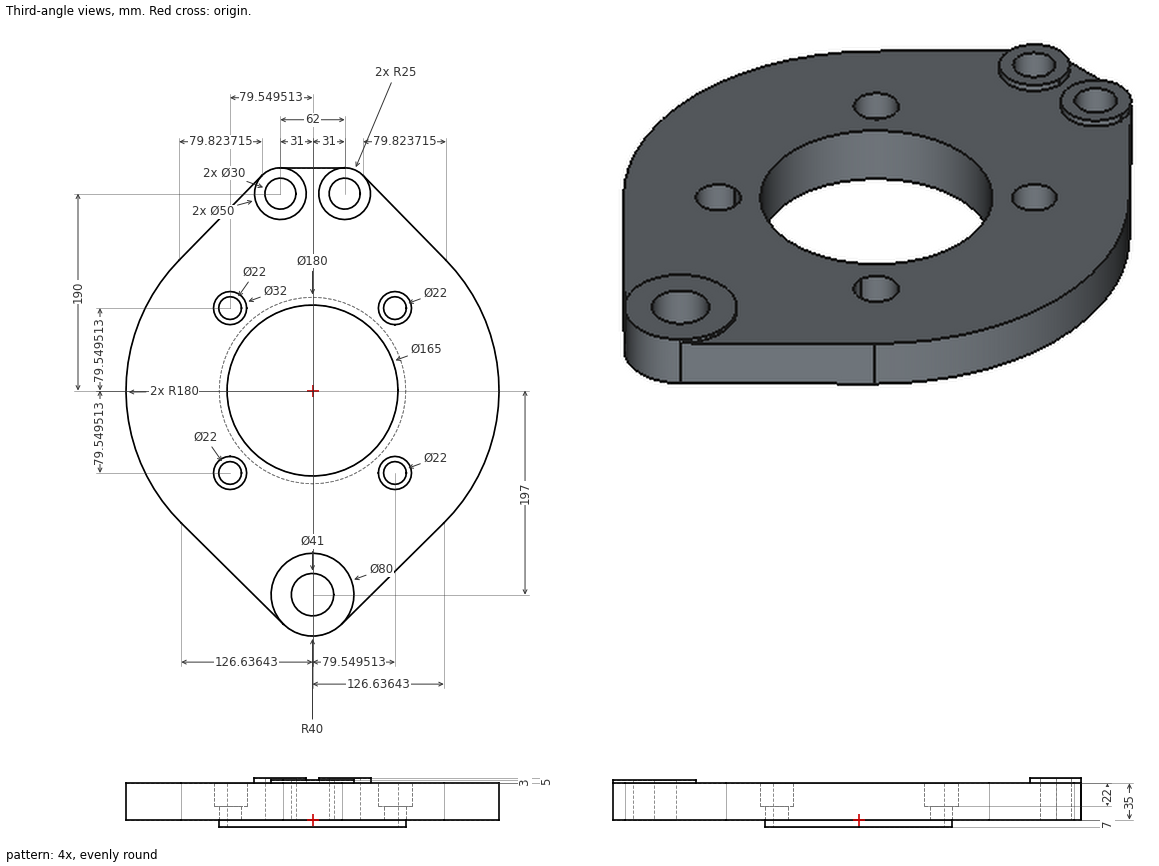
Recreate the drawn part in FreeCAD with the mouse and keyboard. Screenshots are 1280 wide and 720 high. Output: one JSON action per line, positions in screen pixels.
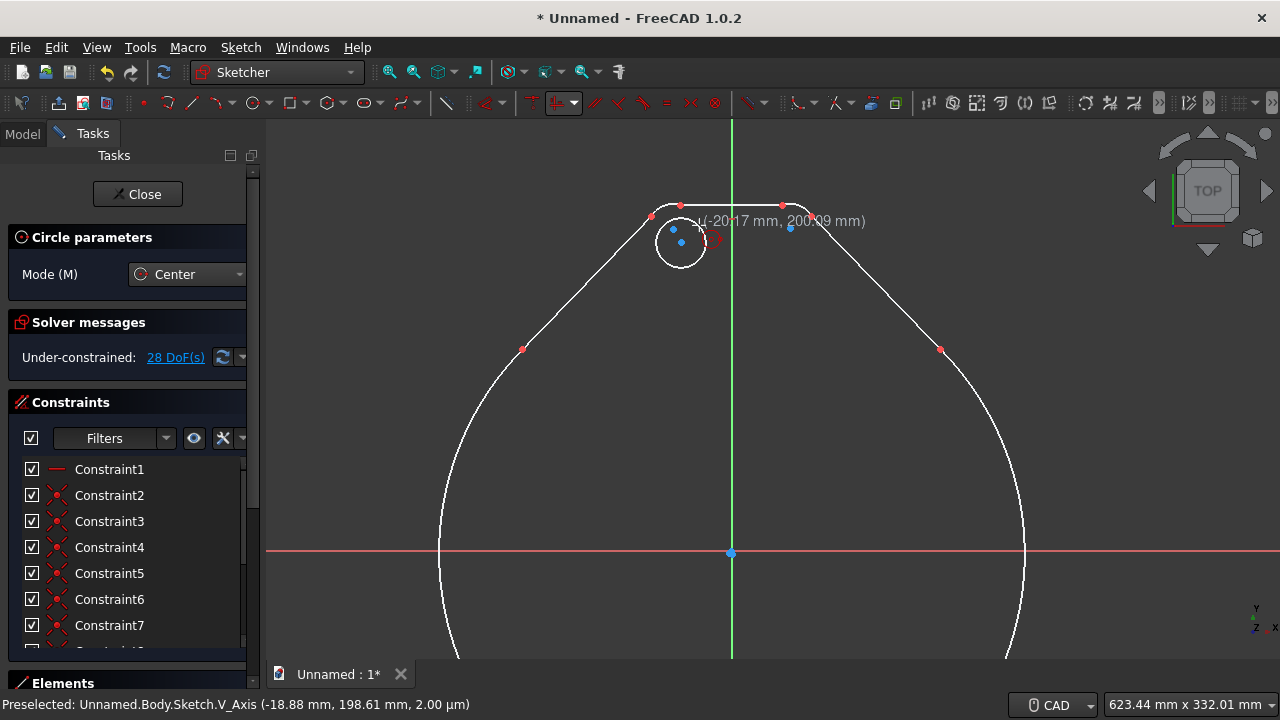
{"action": "left_click", "coordinate": [732, 551]}
{"action": "left_click", "coordinate": [827, 457]}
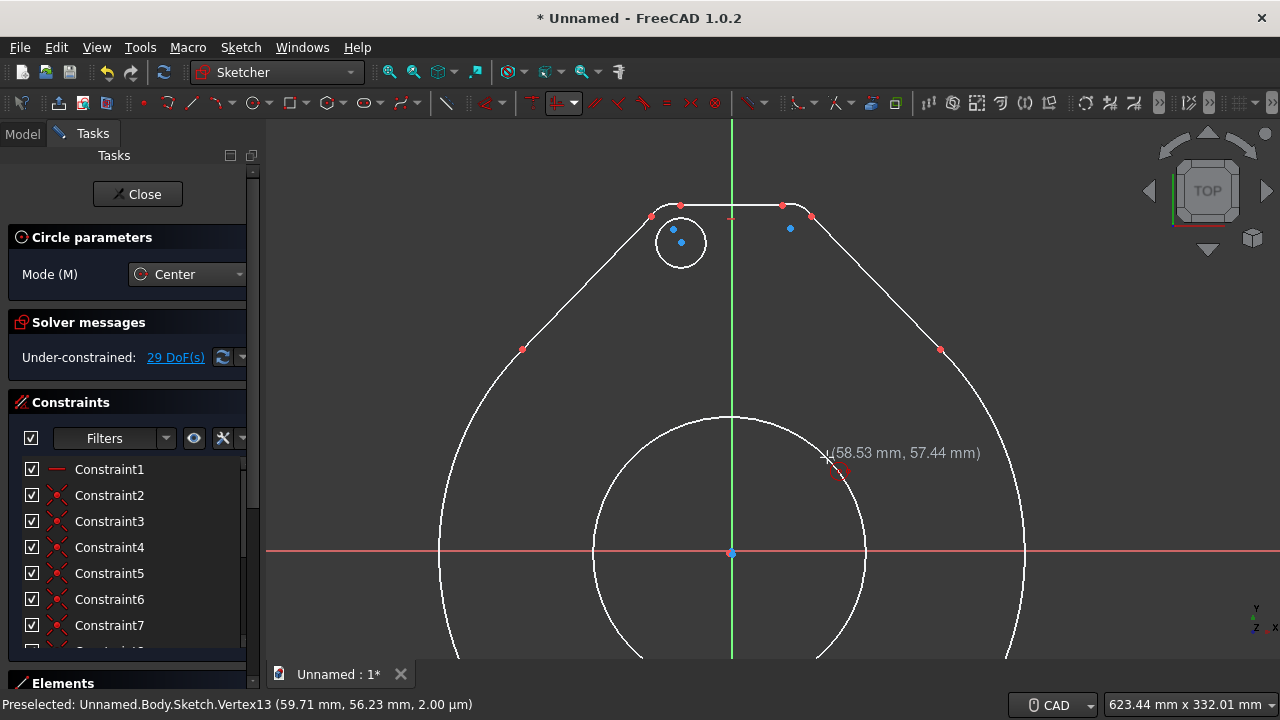
{"action": "left_click", "coordinate": [782, 242]}
{"action": "left_click", "coordinate": [799, 225]}
{"action": "key", "text": "Escape"}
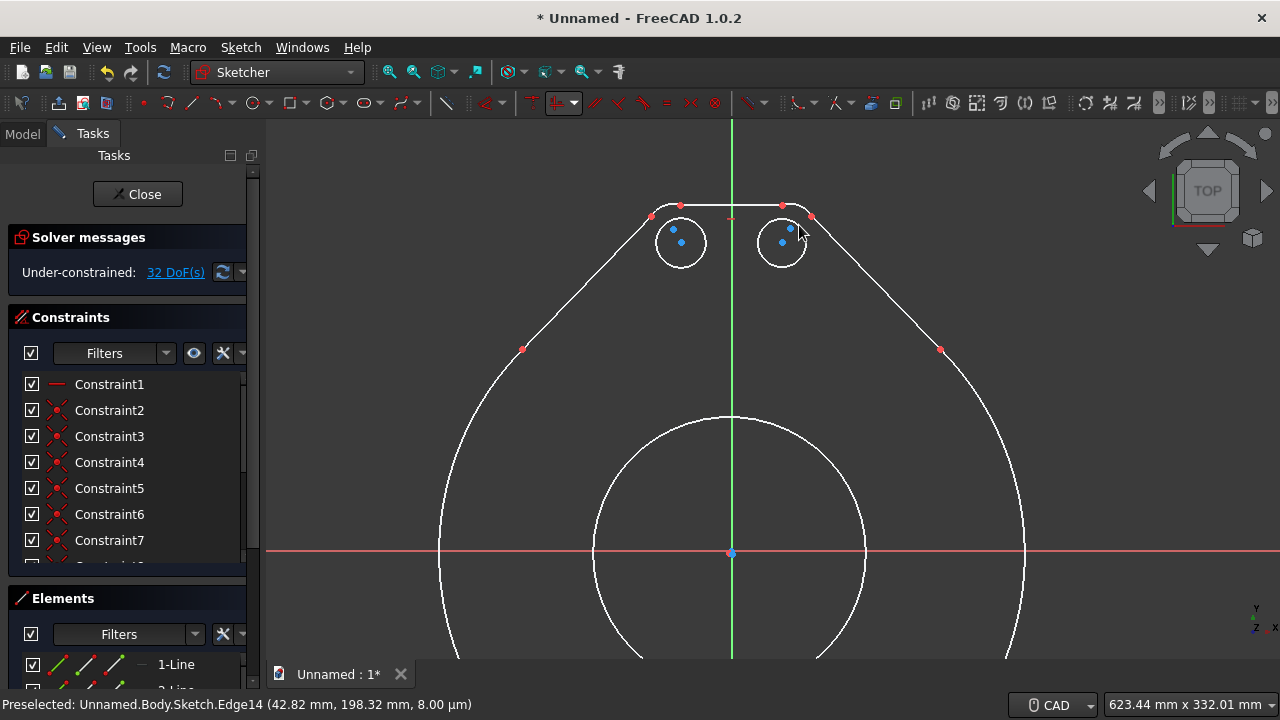
{"action": "left_click", "coordinate": [613, 256]}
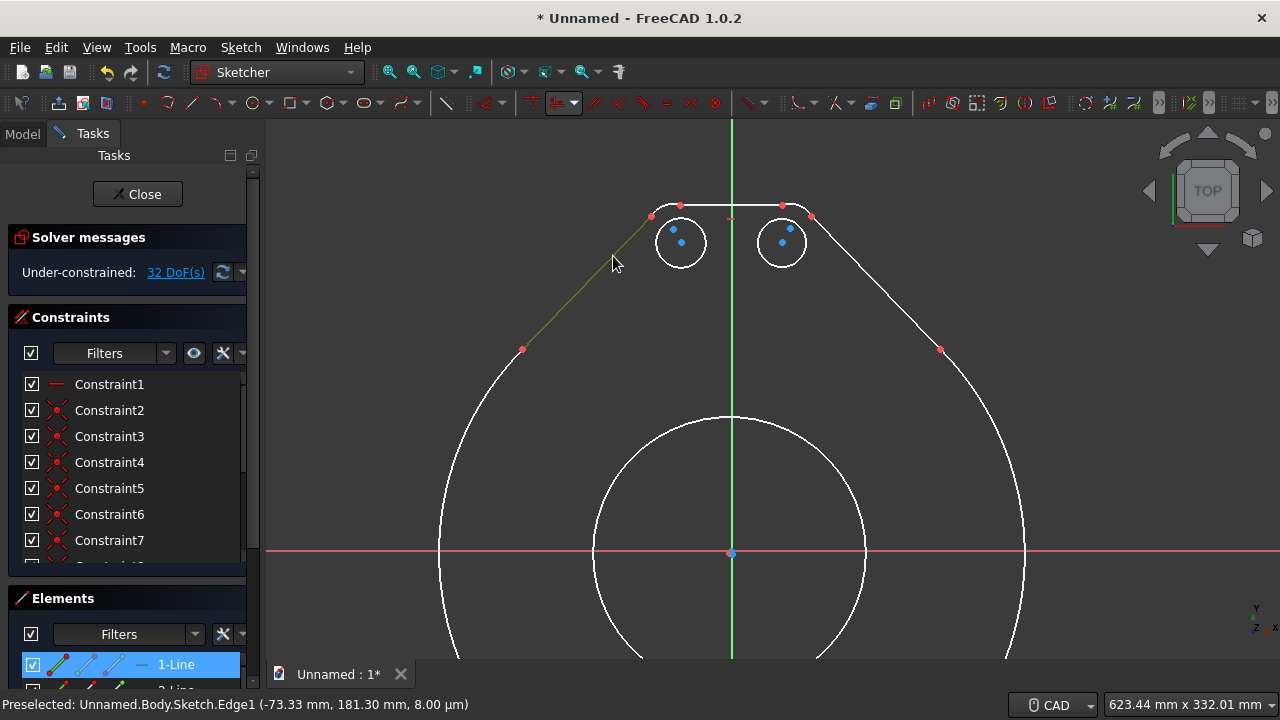
{"action": "scroll", "coordinate": [671, 204], "scroll_direction": "up", "scroll_amount": 2}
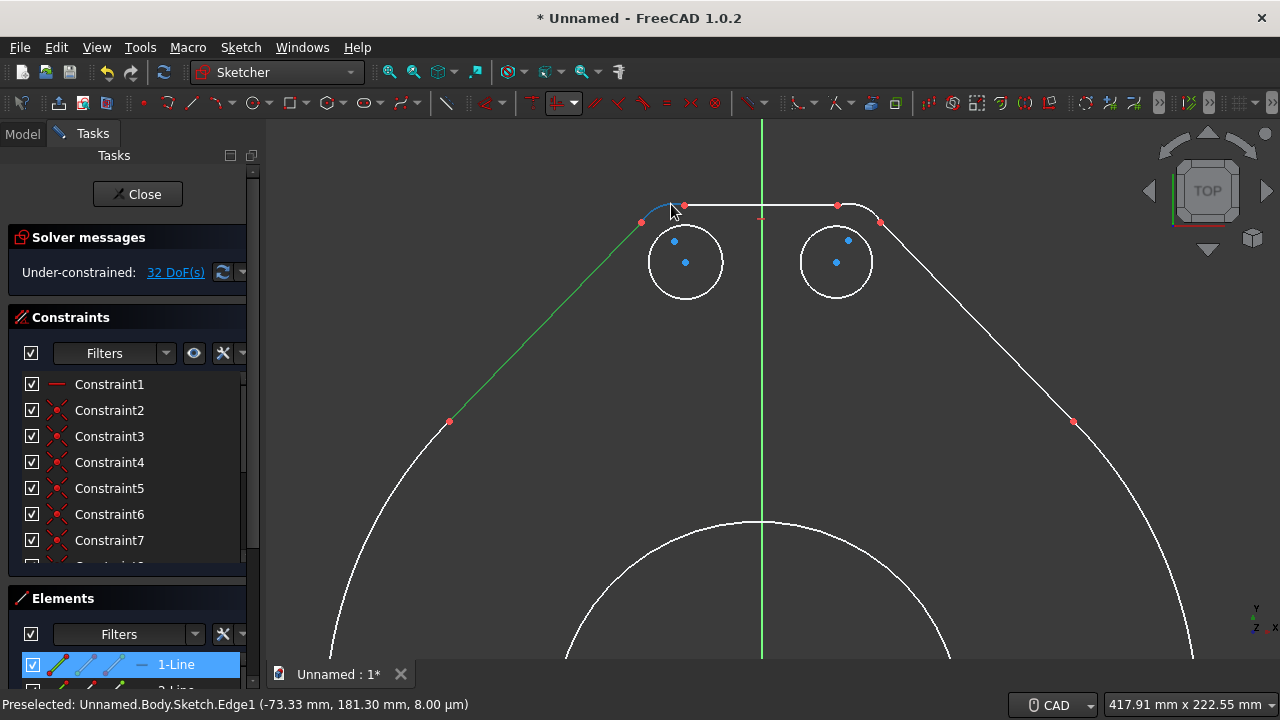
{"action": "left_click", "coordinate": [670, 204]}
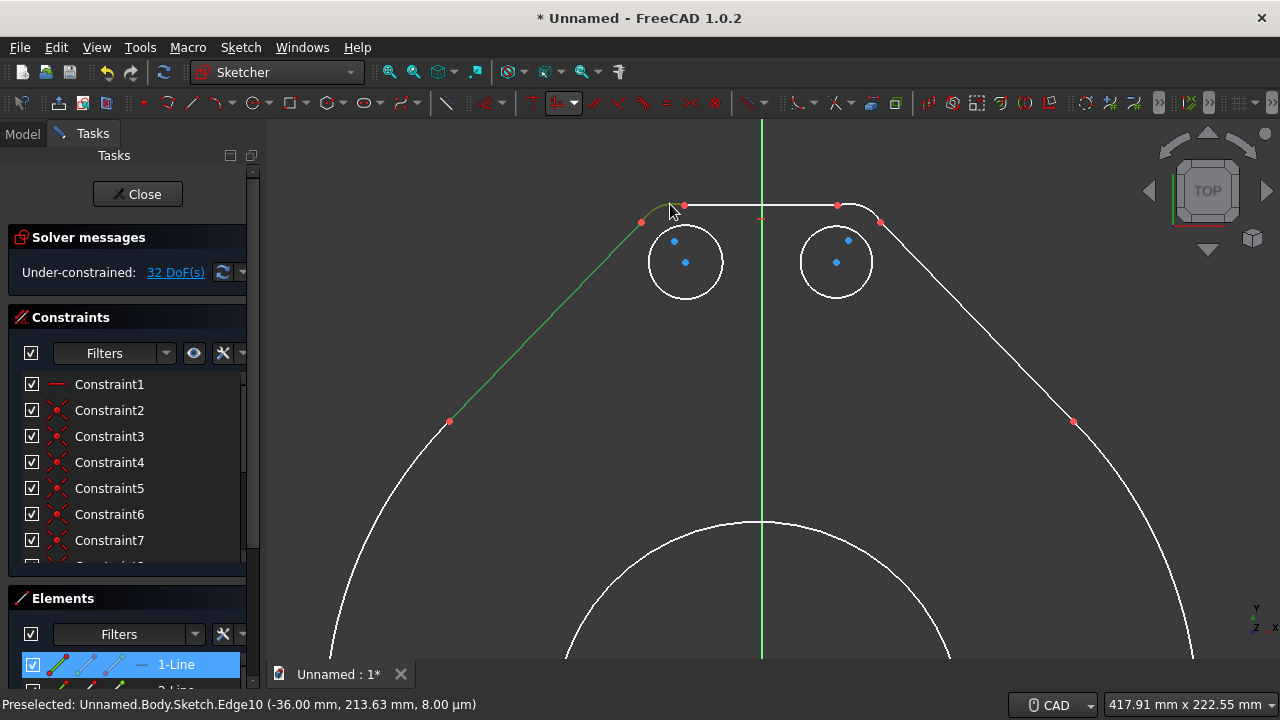
{"action": "left_click", "coordinate": [644, 104]}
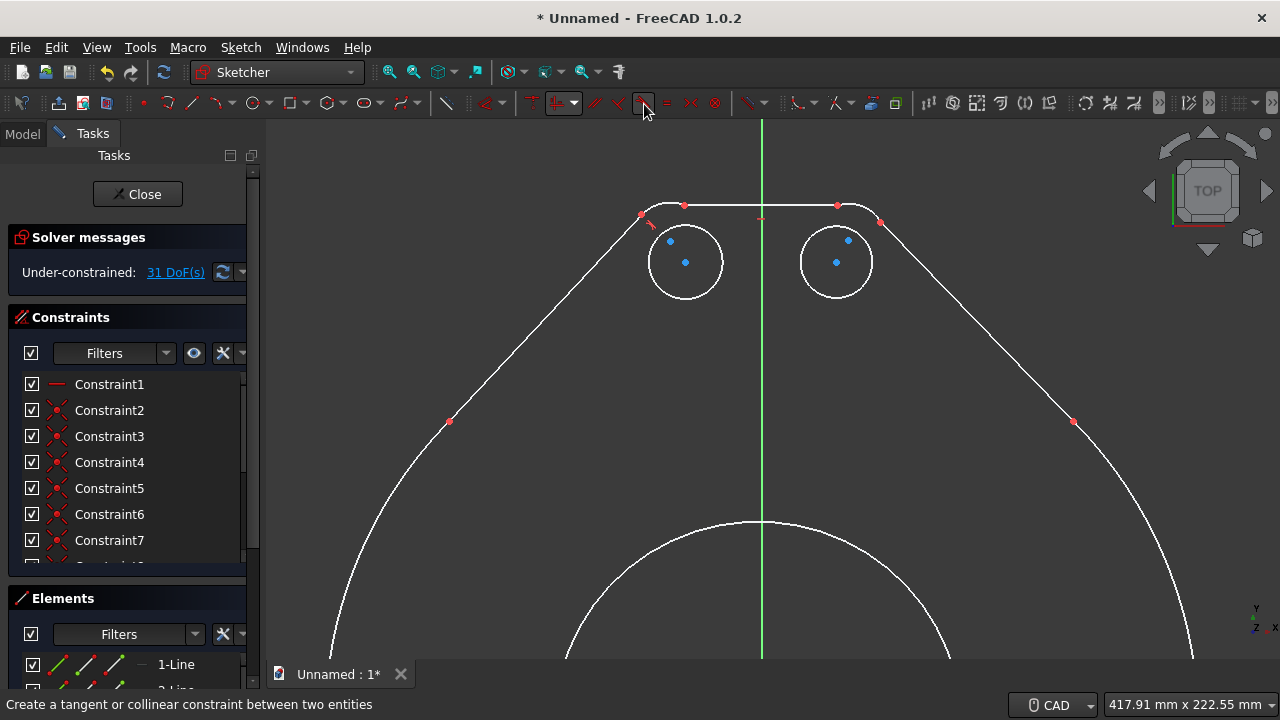
{"action": "scroll", "coordinate": [680, 234], "scroll_direction": "down", "scroll_amount": 6}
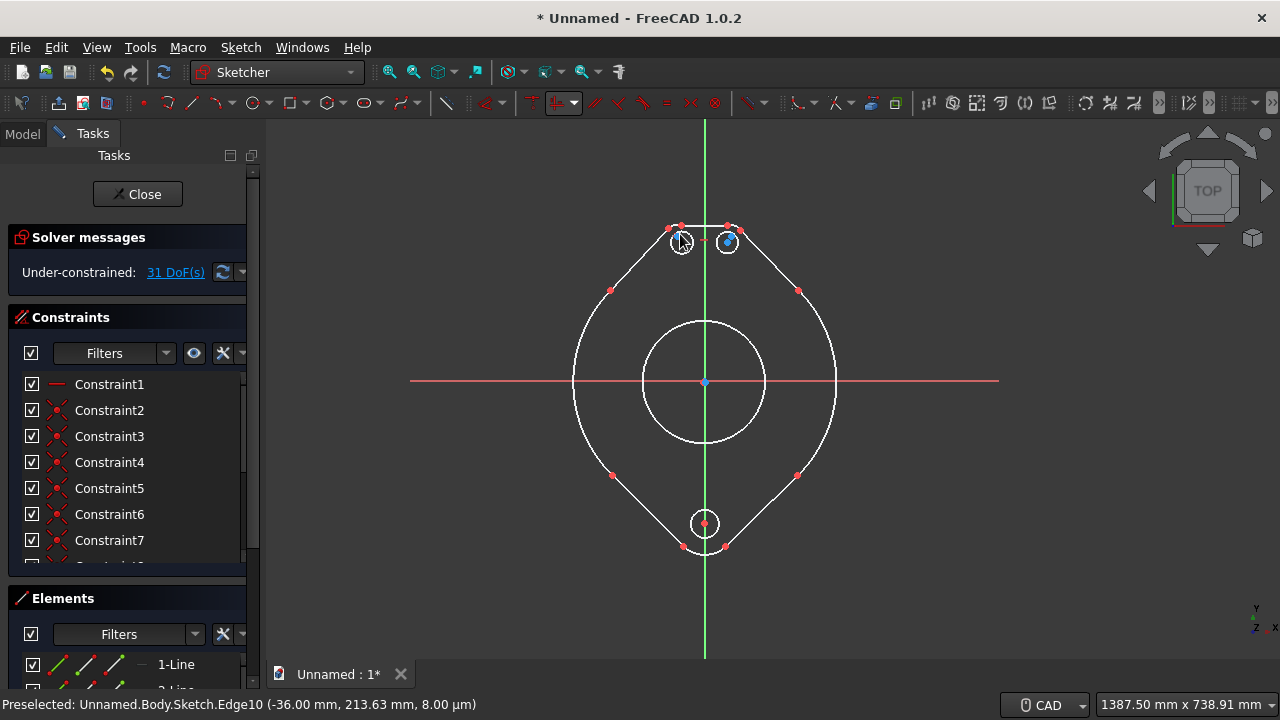
{"action": "left_click", "coordinate": [634, 497]}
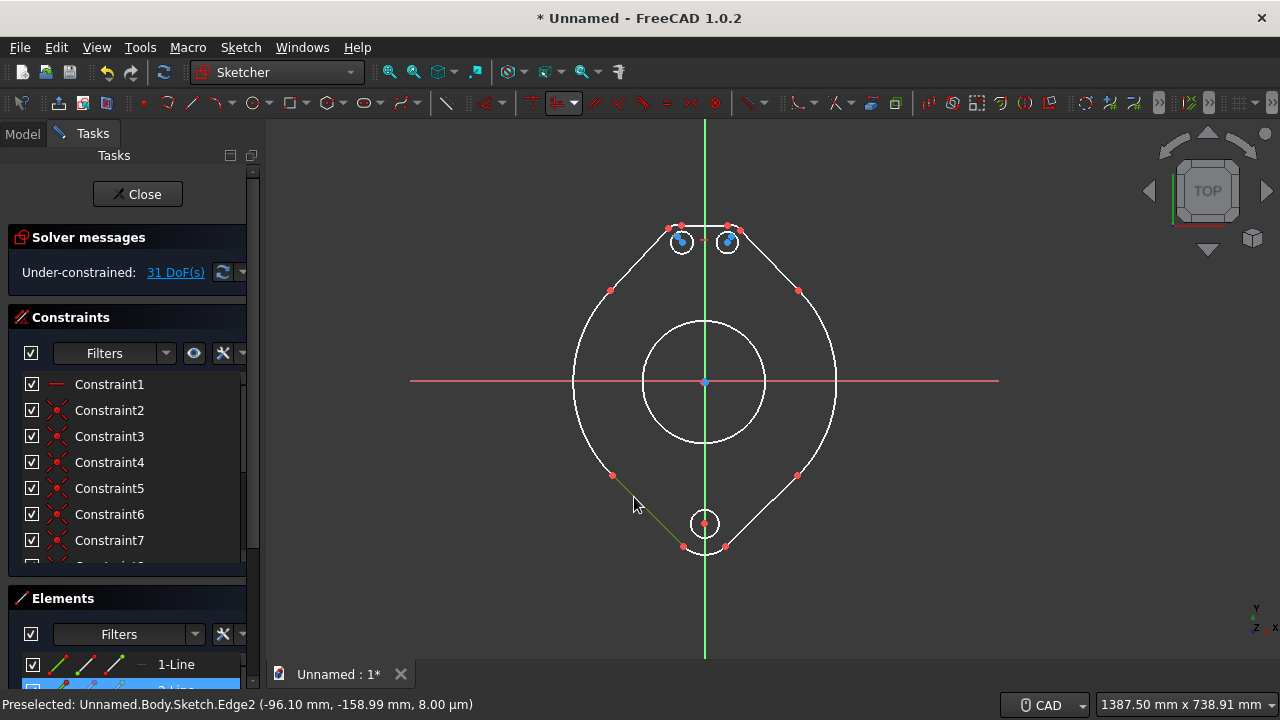
{"action": "scroll", "coordinate": [696, 553], "scroll_direction": "up", "scroll_amount": 3}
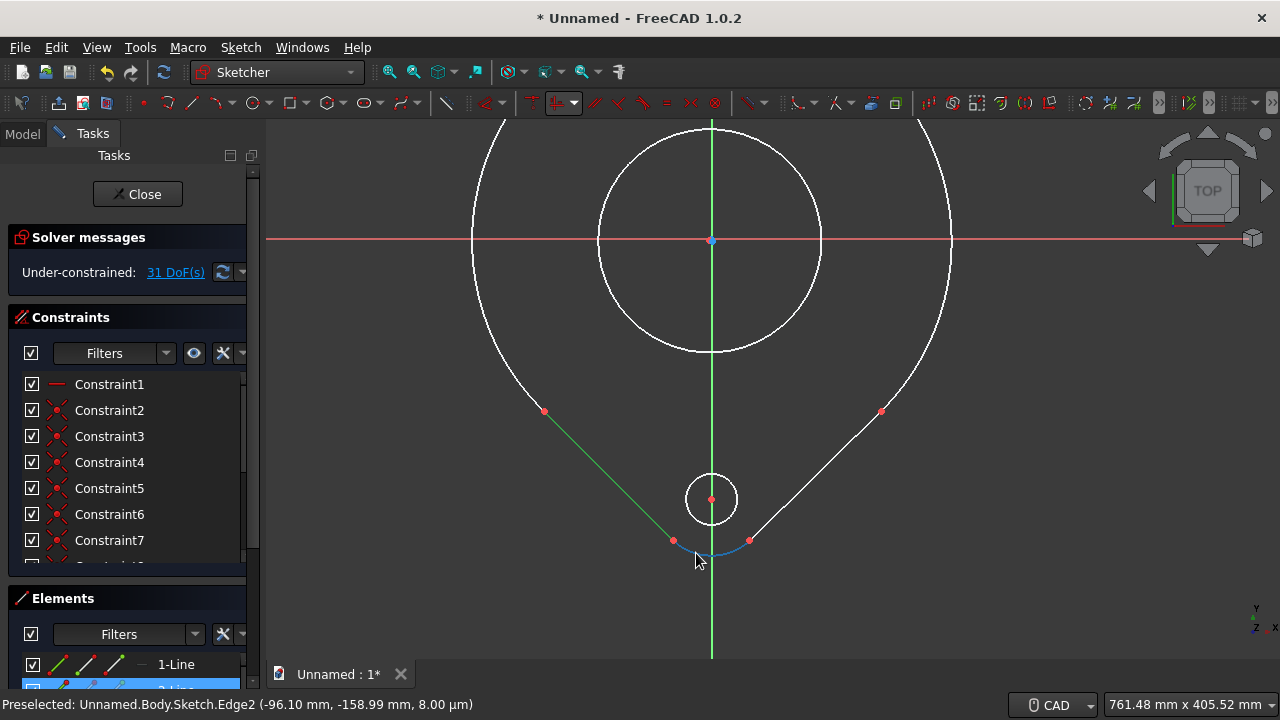
{"action": "left_click", "coordinate": [695, 553]}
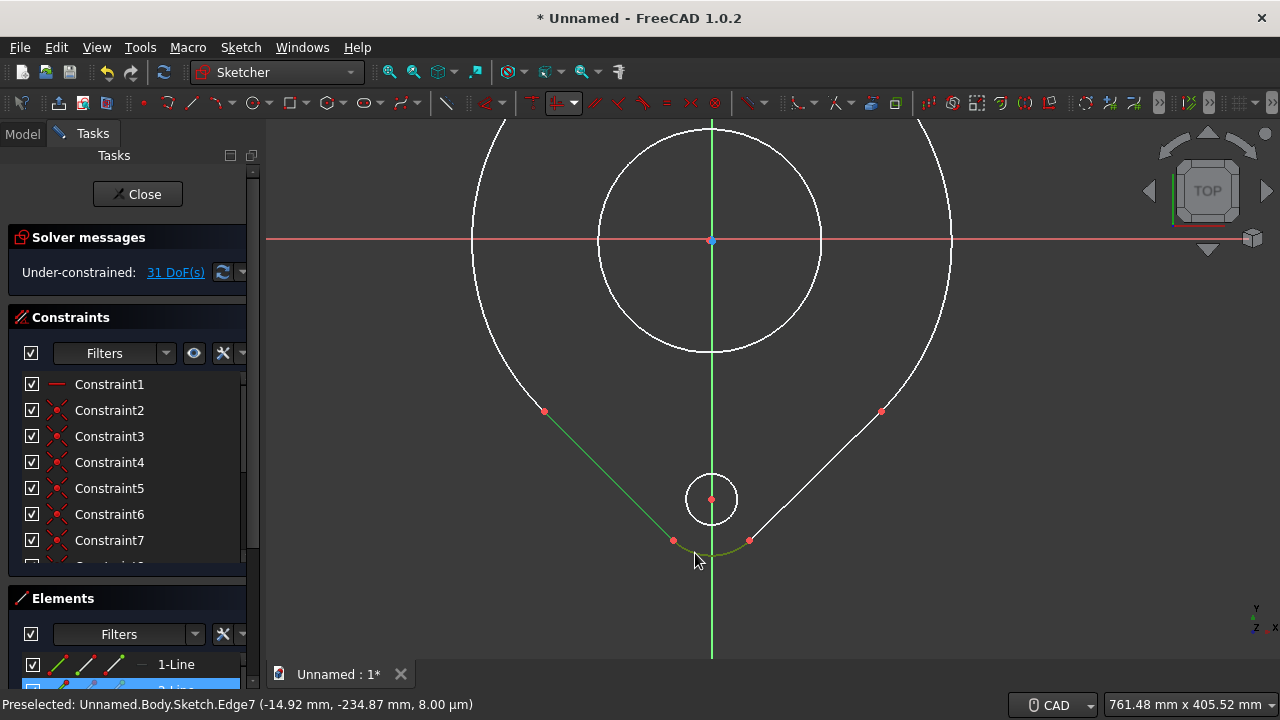
{"action": "key", "text": "t"}